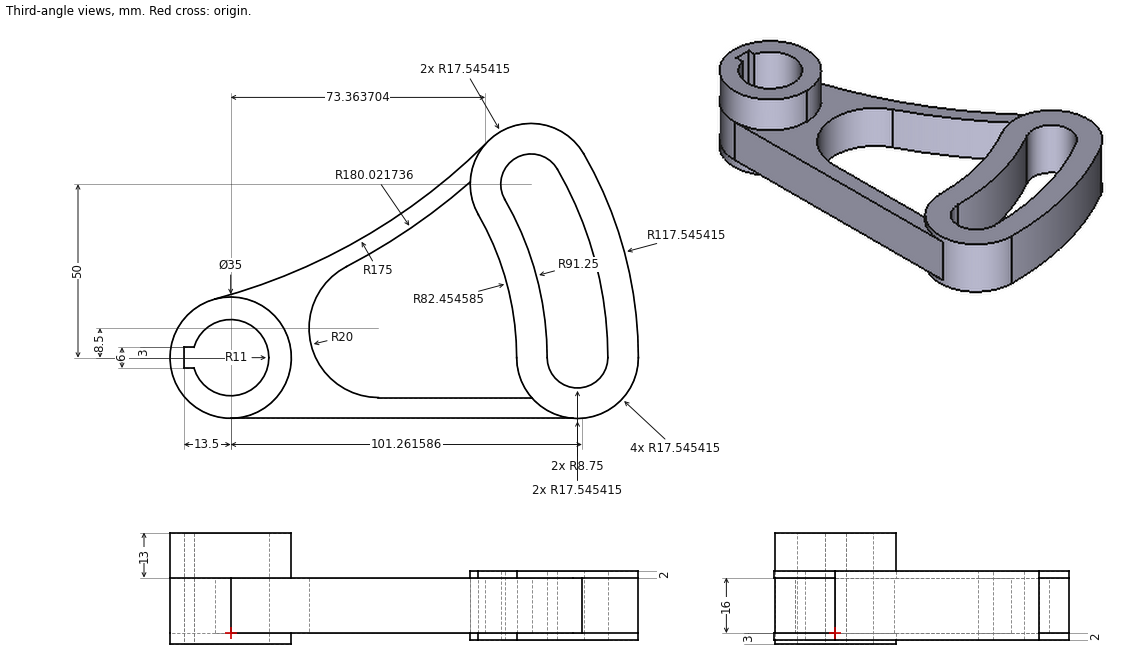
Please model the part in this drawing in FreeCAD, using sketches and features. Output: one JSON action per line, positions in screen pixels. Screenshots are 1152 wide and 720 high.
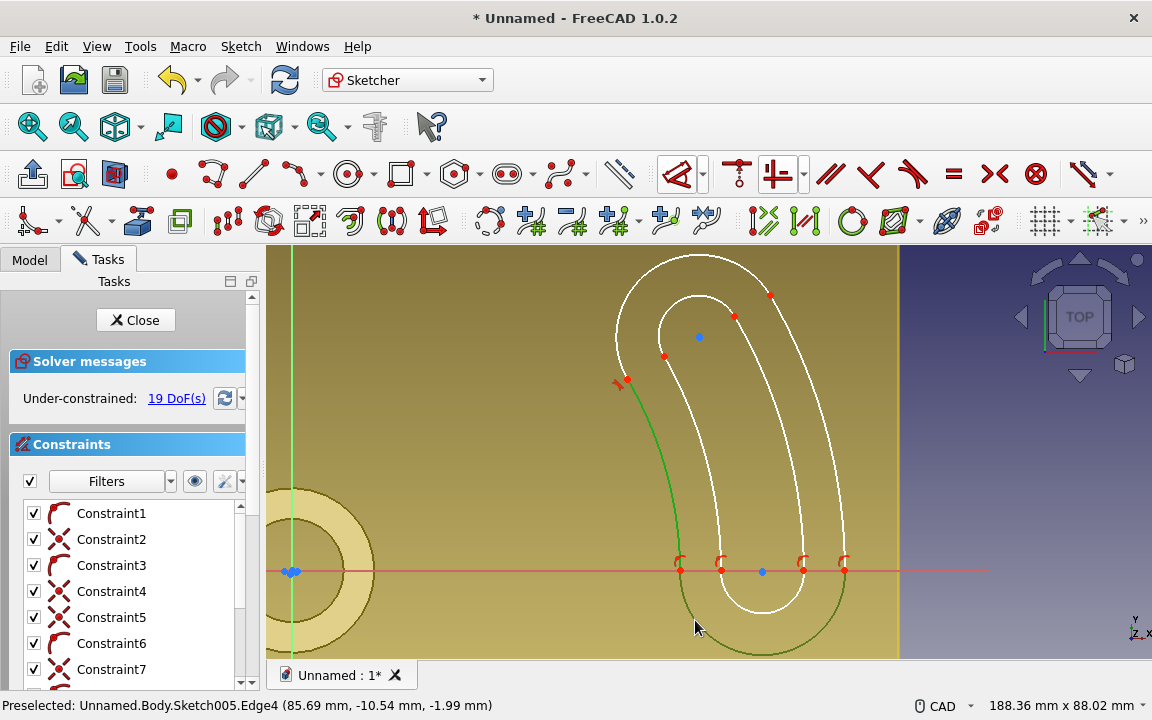
{"action": "left_click", "coordinate": [913, 174]}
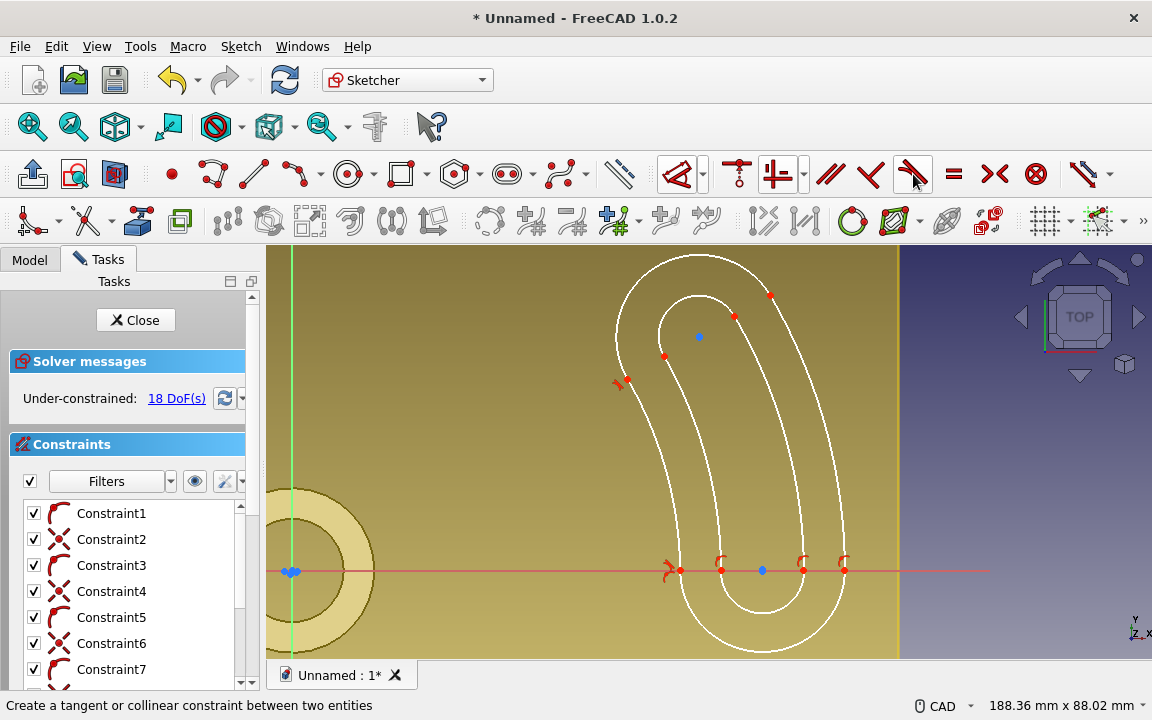
{"action": "left_click", "coordinate": [623, 304]}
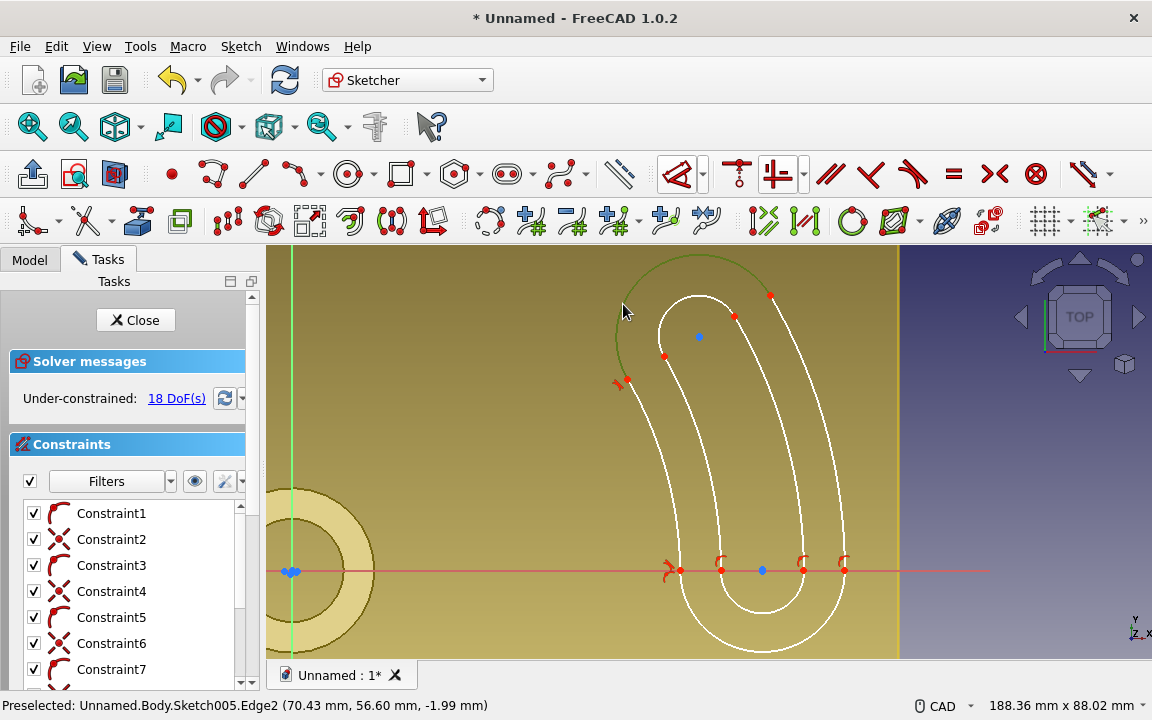
{"action": "left_click", "coordinate": [838, 484]}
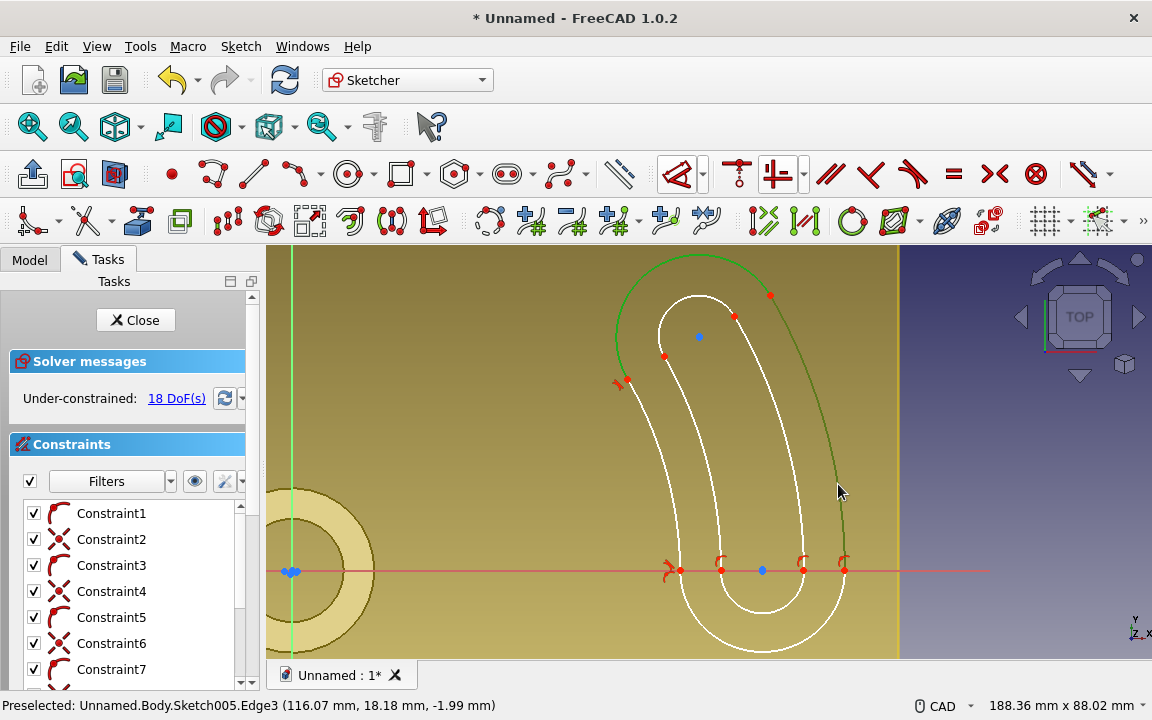
{"action": "left_click", "coordinate": [913, 174]}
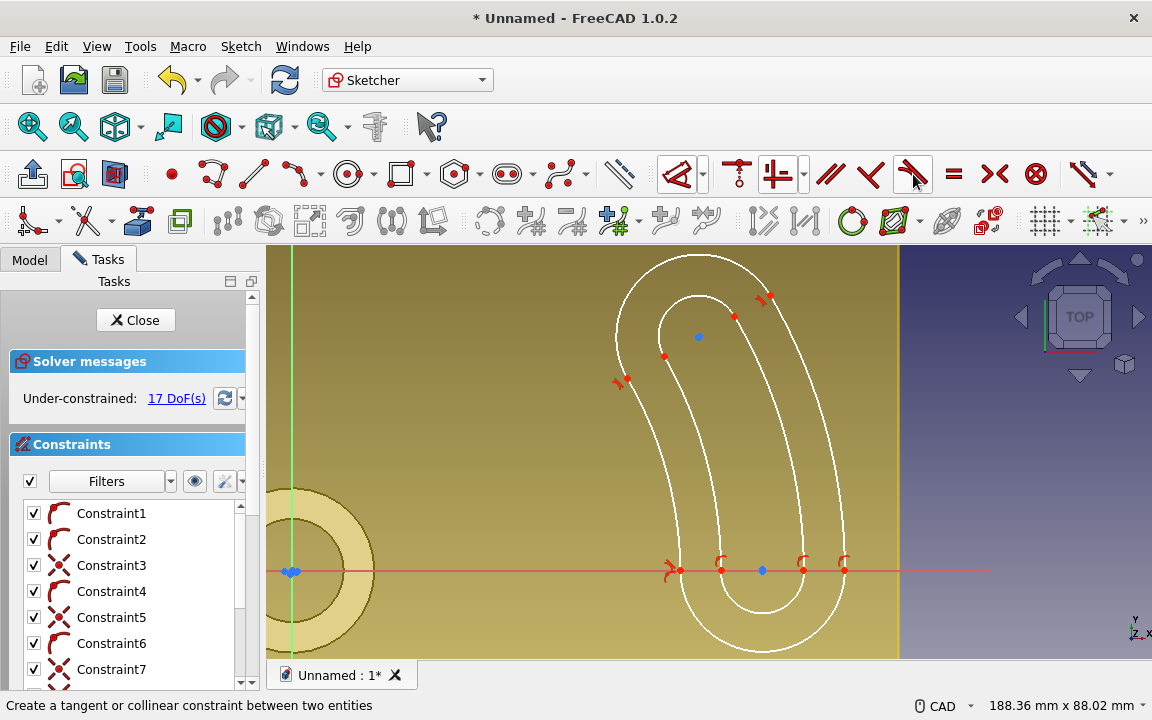
{"action": "left_click", "coordinate": [716, 504]}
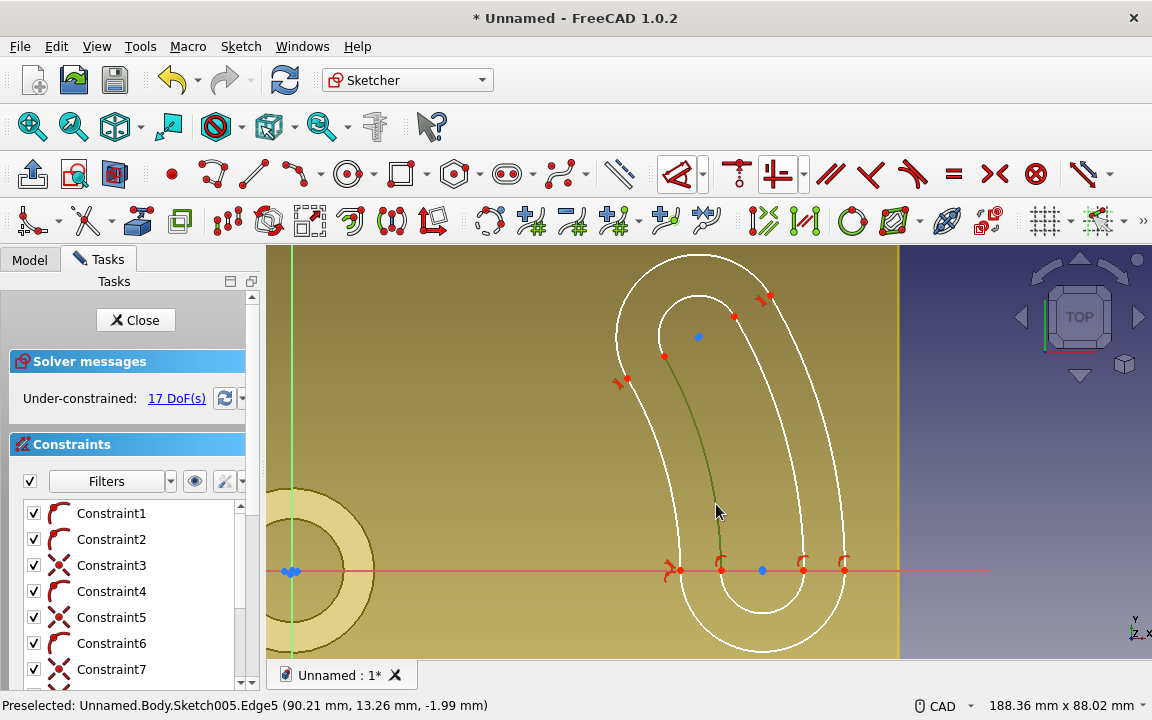
{"action": "left_click", "coordinate": [738, 605]}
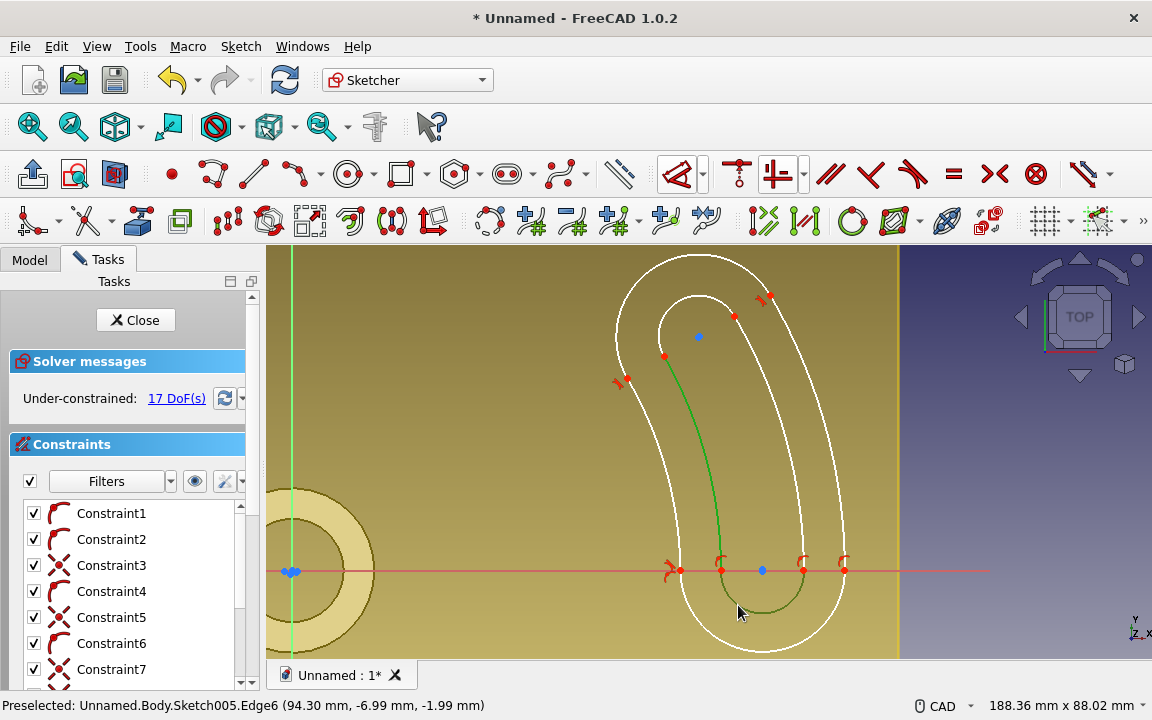
{"action": "left_click", "coordinate": [913, 174]}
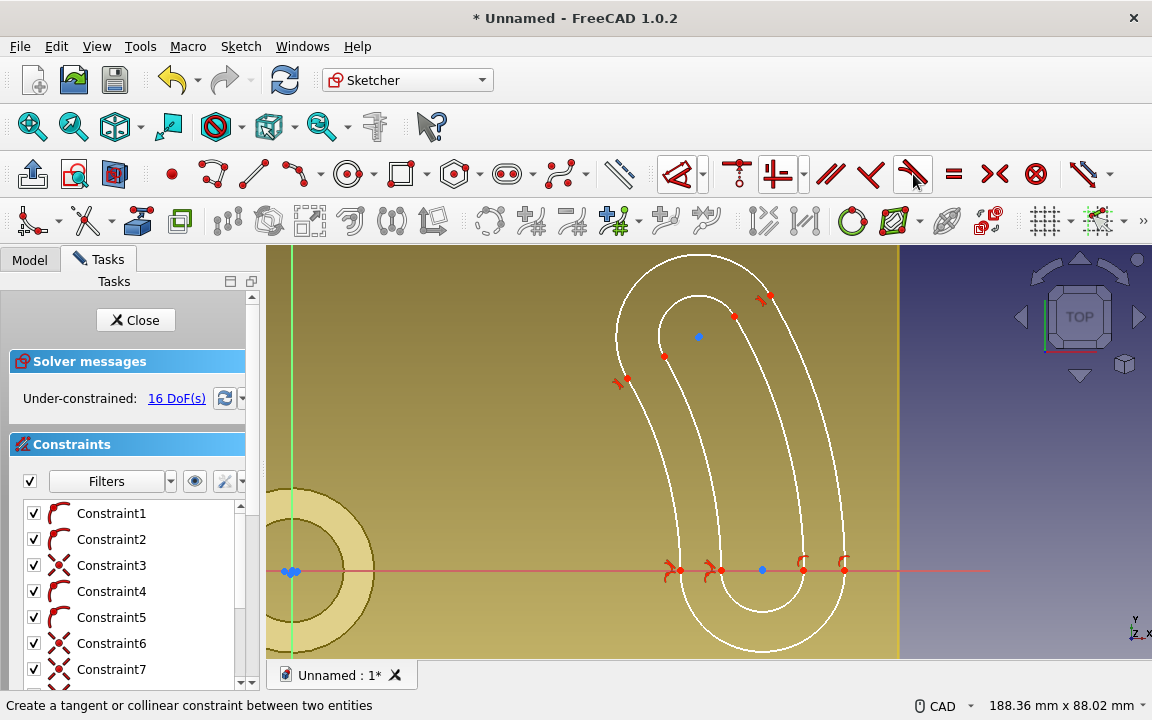
{"action": "left_click", "coordinate": [716, 504]}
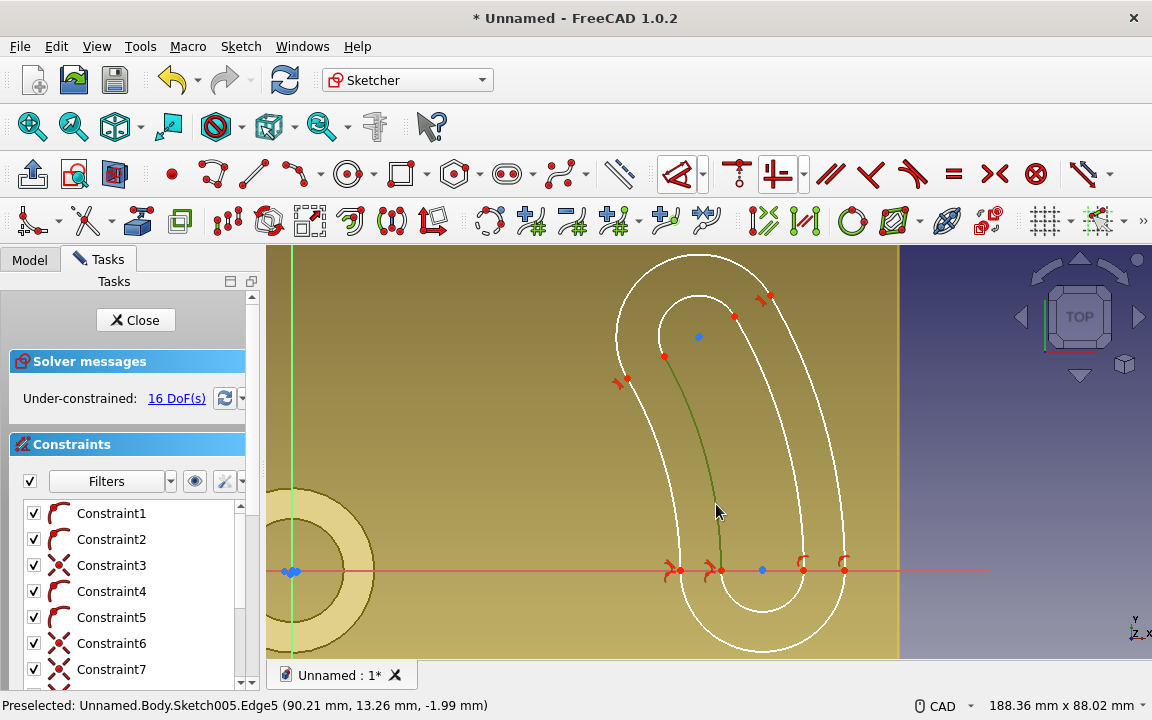
{"action": "left_click", "coordinate": [704, 296]}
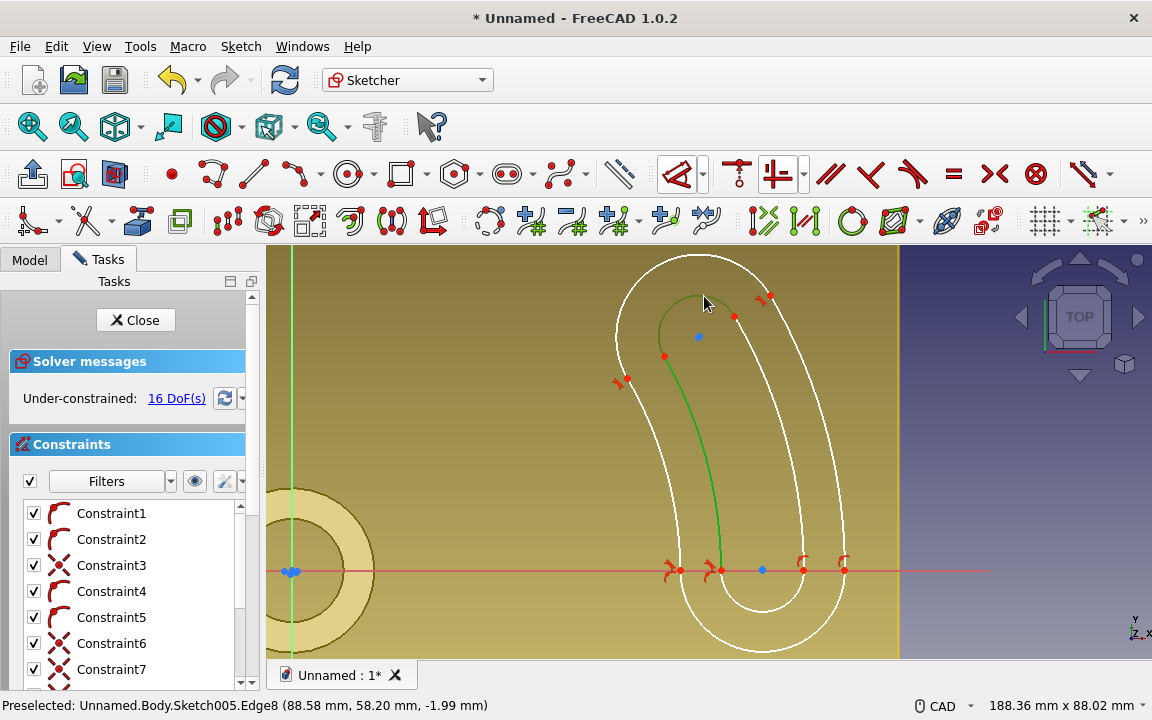
{"action": "left_click", "coordinate": [913, 174]}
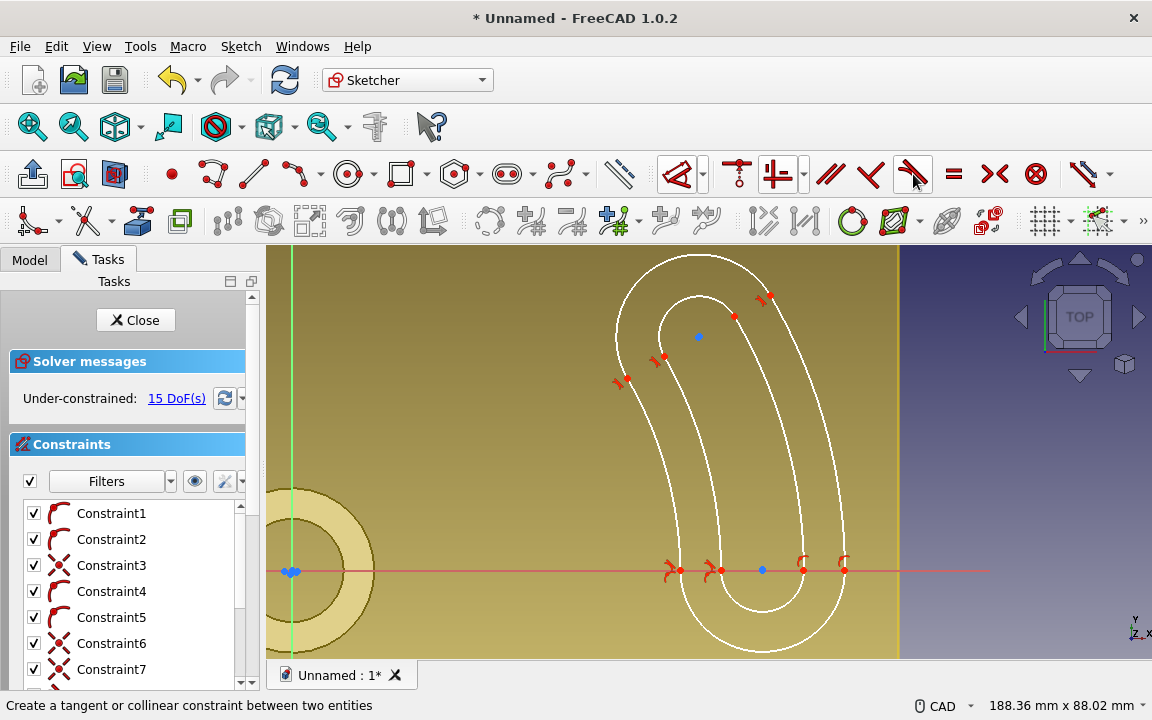
{"action": "left_click", "coordinate": [797, 491]}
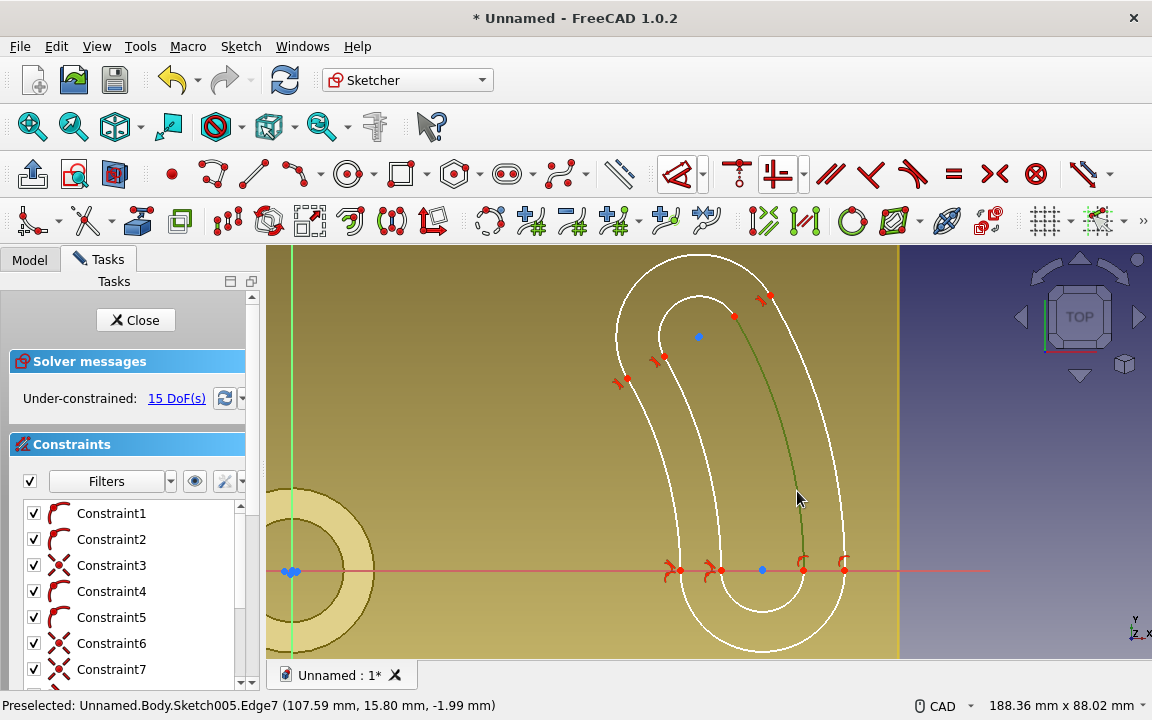
{"action": "left_click", "coordinate": [704, 297]}